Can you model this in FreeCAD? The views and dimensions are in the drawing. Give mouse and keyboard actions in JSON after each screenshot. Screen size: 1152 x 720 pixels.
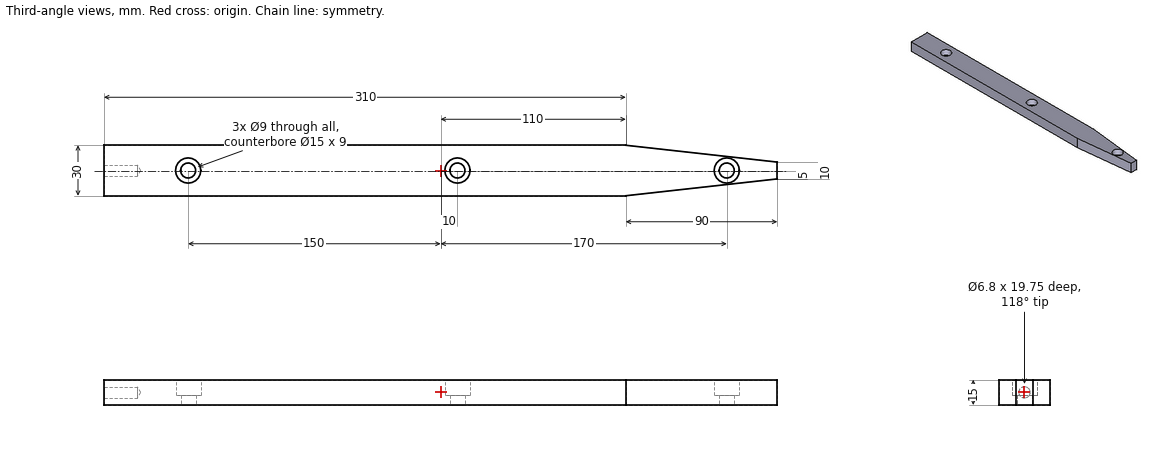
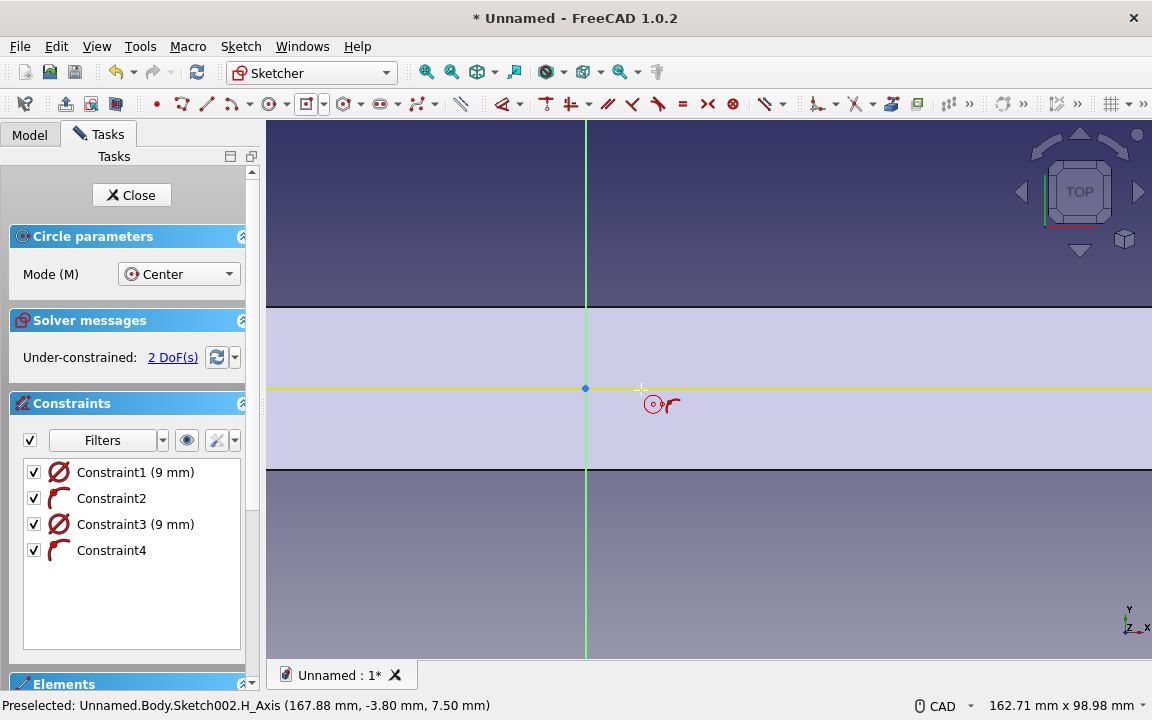
{"action": "scroll", "coordinate": [641, 390], "scroll_direction": "down", "scroll_amount": 6}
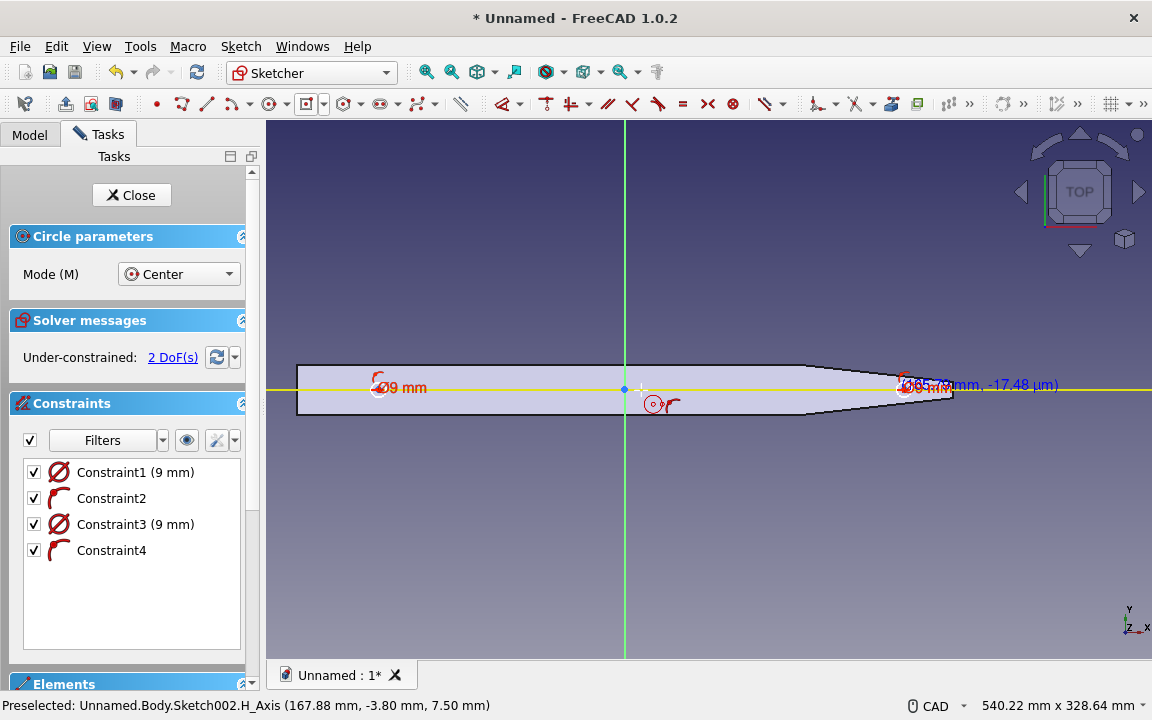
{"action": "left_click", "coordinate": [641, 390]}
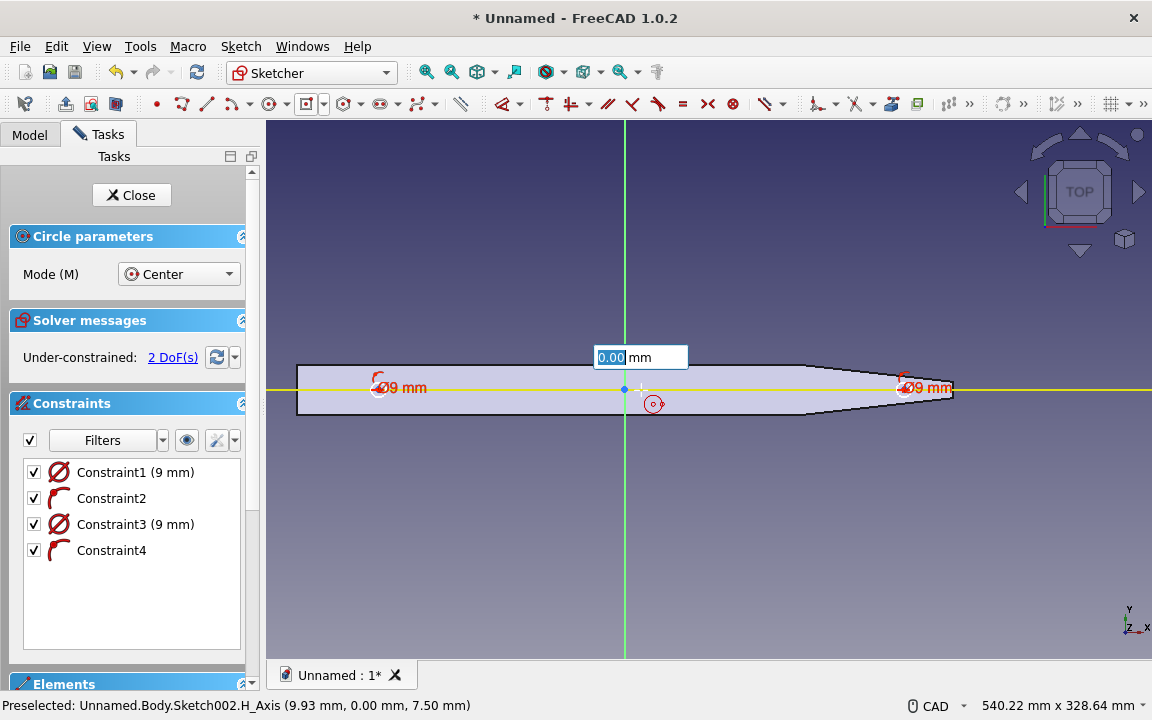
{"action": "scroll", "coordinate": [639, 397], "scroll_direction": "up", "scroll_amount": 5}
{"action": "mouse_move", "coordinate": [637, 396]}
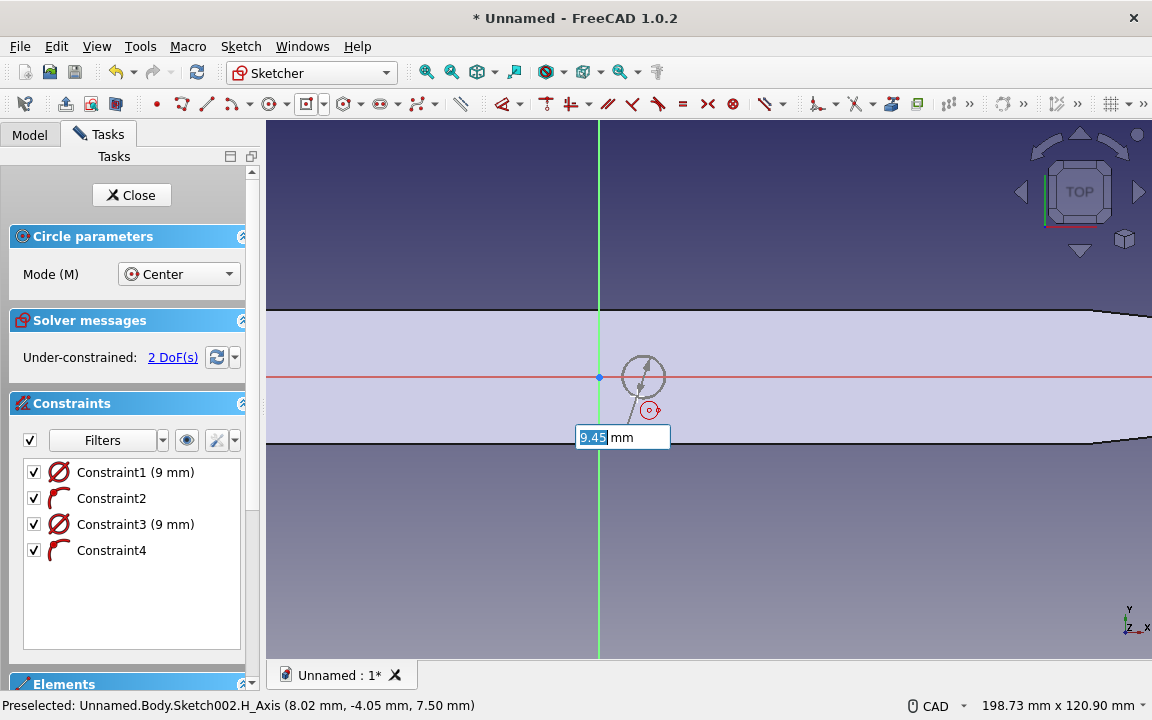
{"action": "type", "text": "9"}
{"action": "key", "text": "Return"}
{"action": "key", "text": "Escape"}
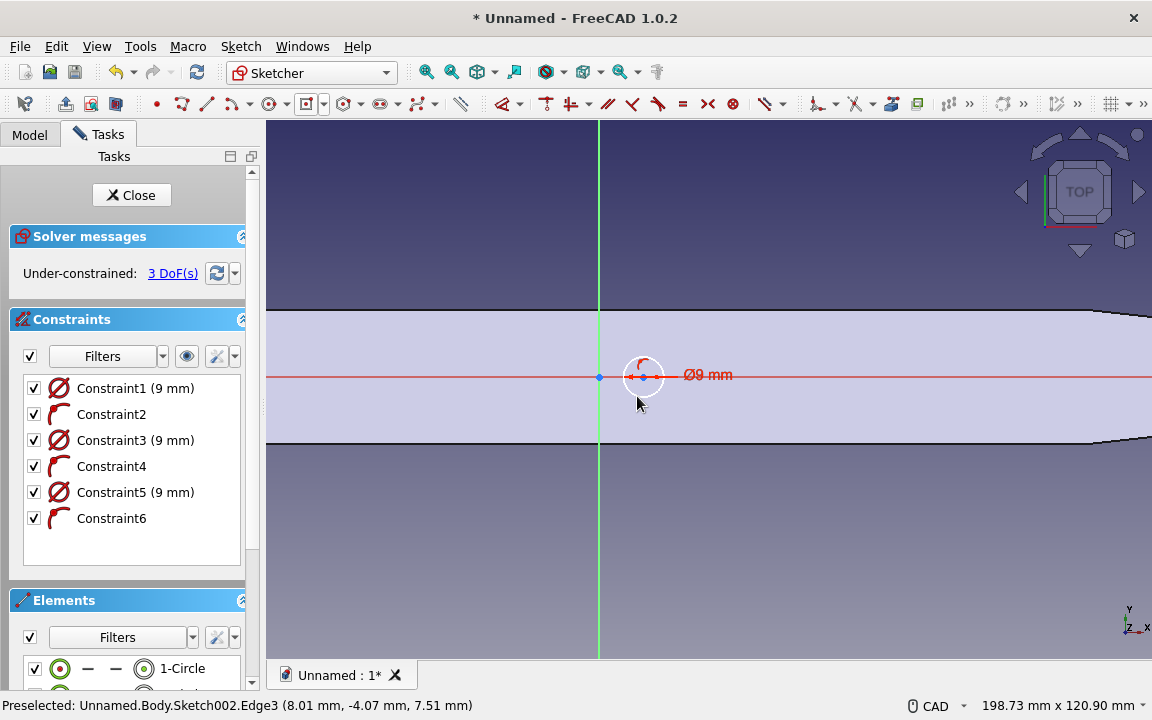
{"action": "key", "text": "d"}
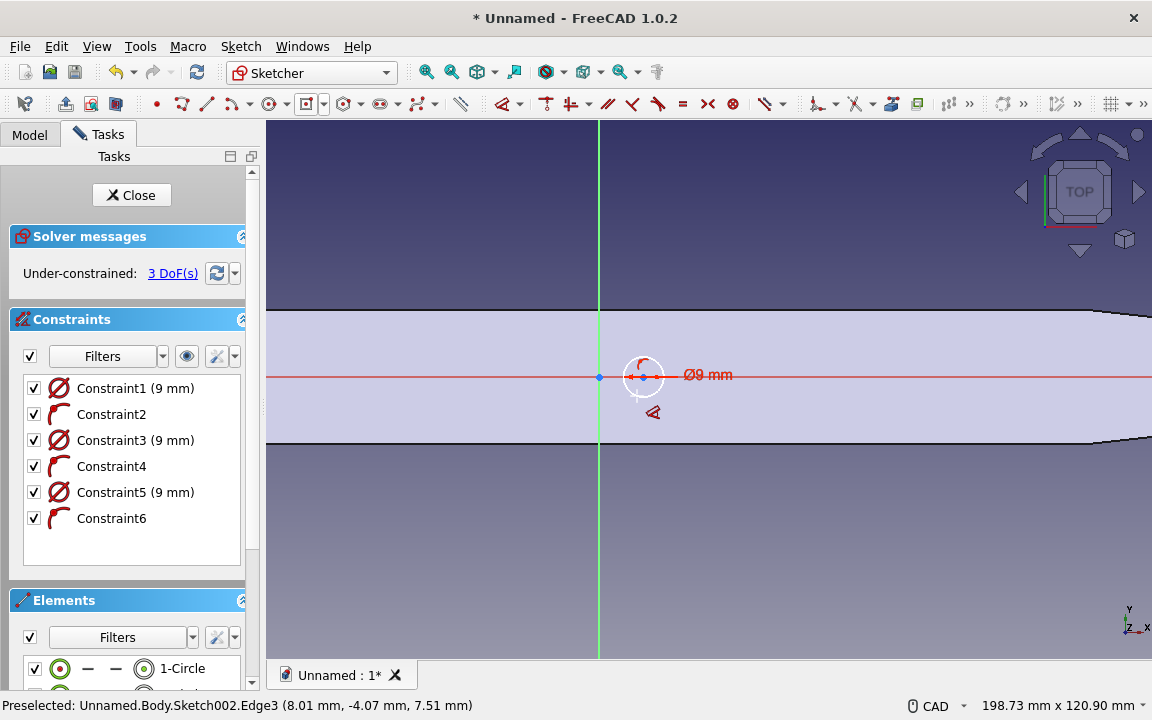
{"action": "left_click", "coordinate": [644, 377]}
{"action": "left_click", "coordinate": [622, 411]}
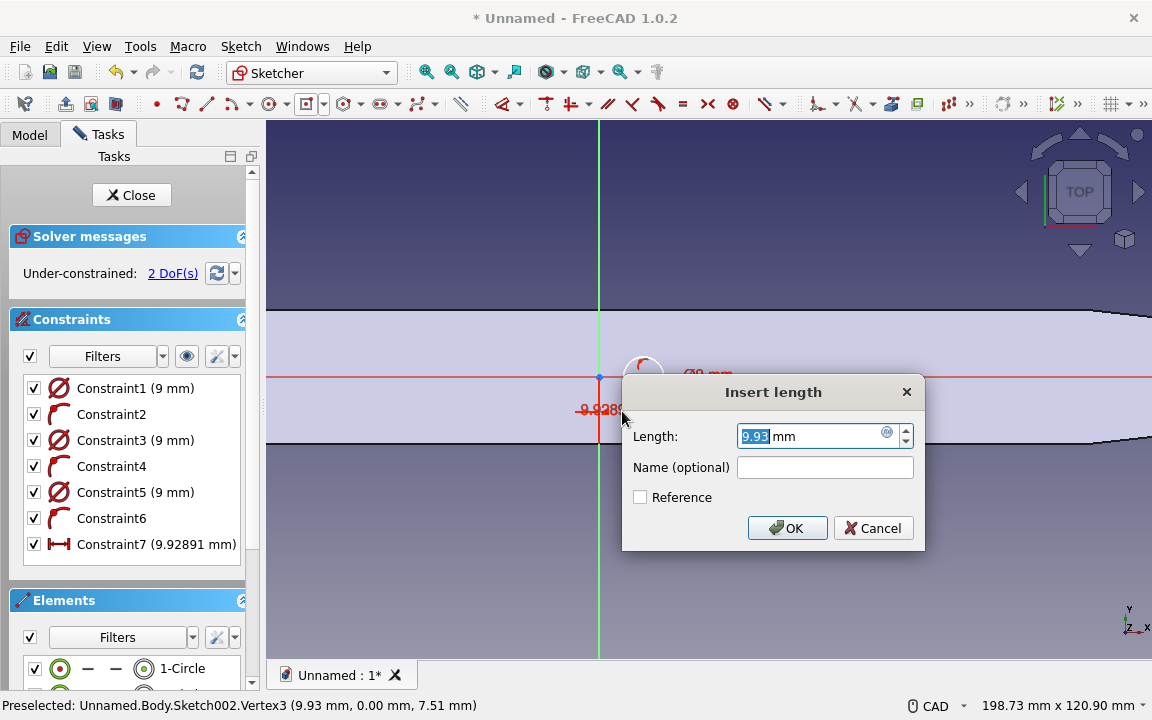
{"action": "type", "text": "10"}
{"action": "key", "text": "Return"}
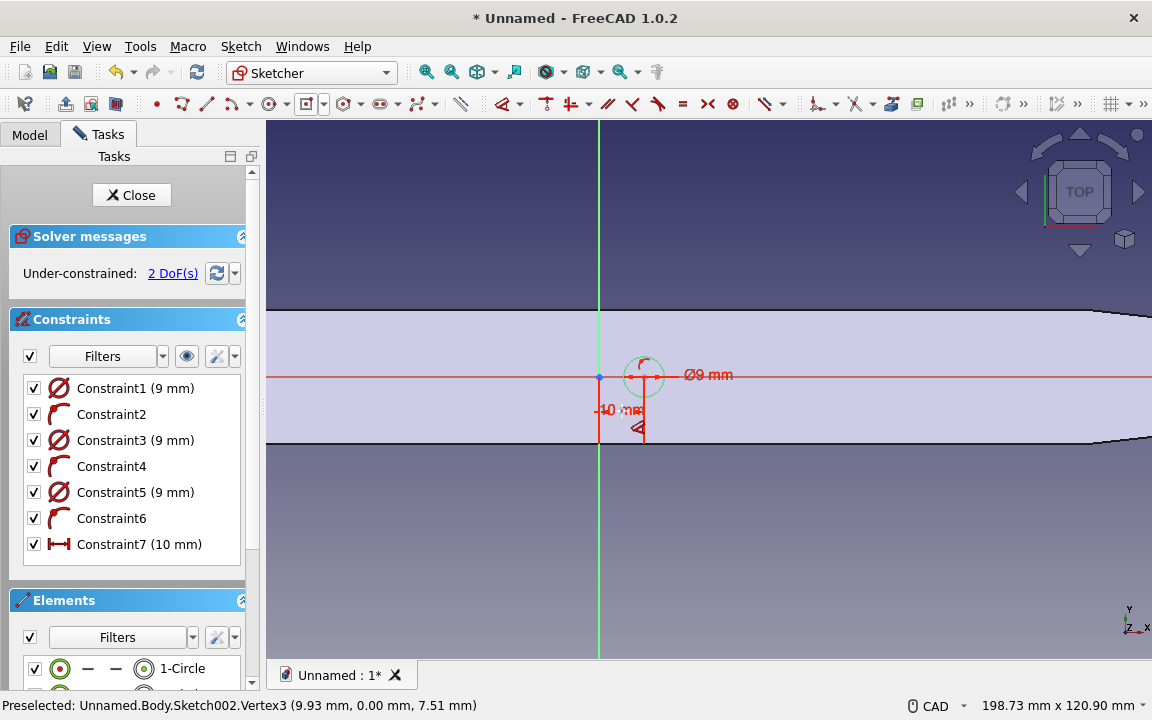
{"action": "scroll", "coordinate": [638, 397], "scroll_direction": "down", "scroll_amount": 5}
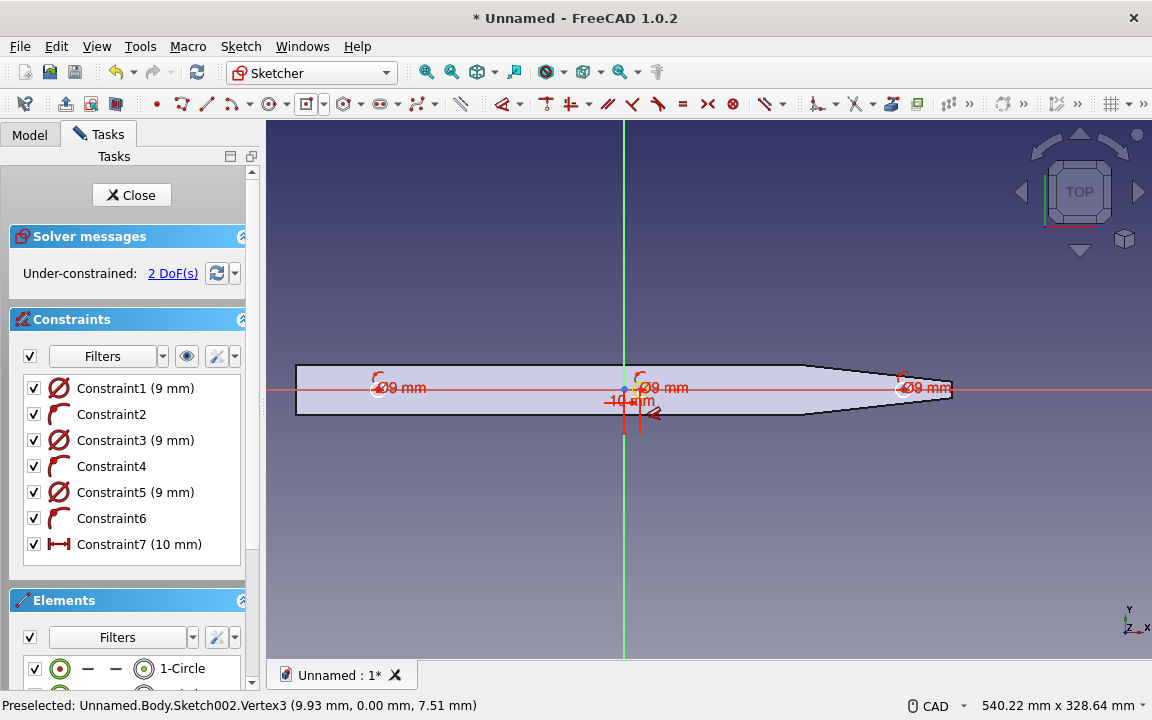
{"action": "left_click", "coordinate": [378, 390]}
{"action": "left_click", "coordinate": [501, 424]}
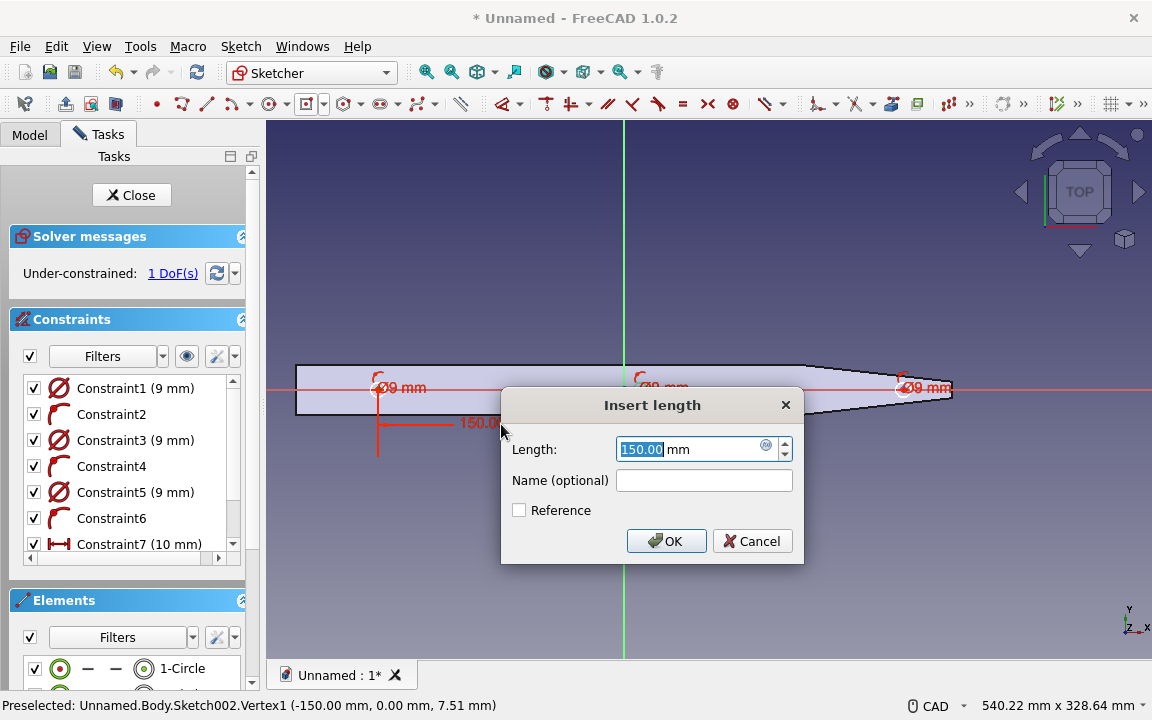
{"action": "type", "text": "150"}
{"action": "key", "text": "Return"}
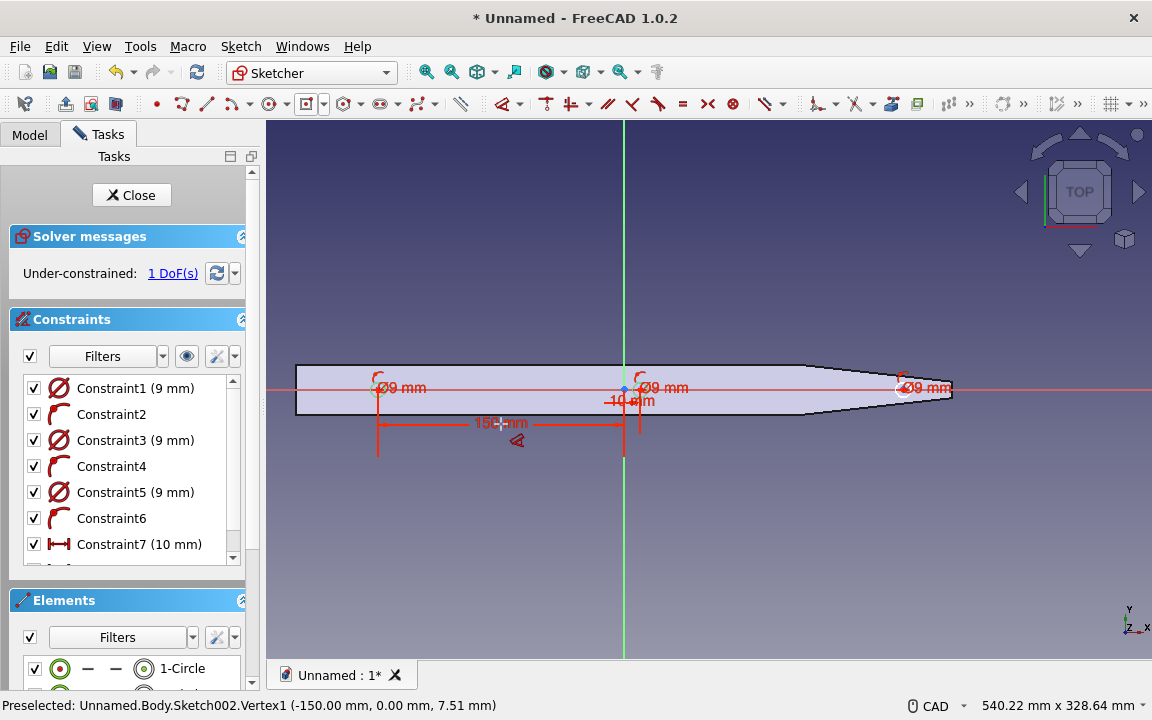
{"action": "left_click", "coordinate": [903, 390]}
{"action": "left_click", "coordinate": [764, 424]}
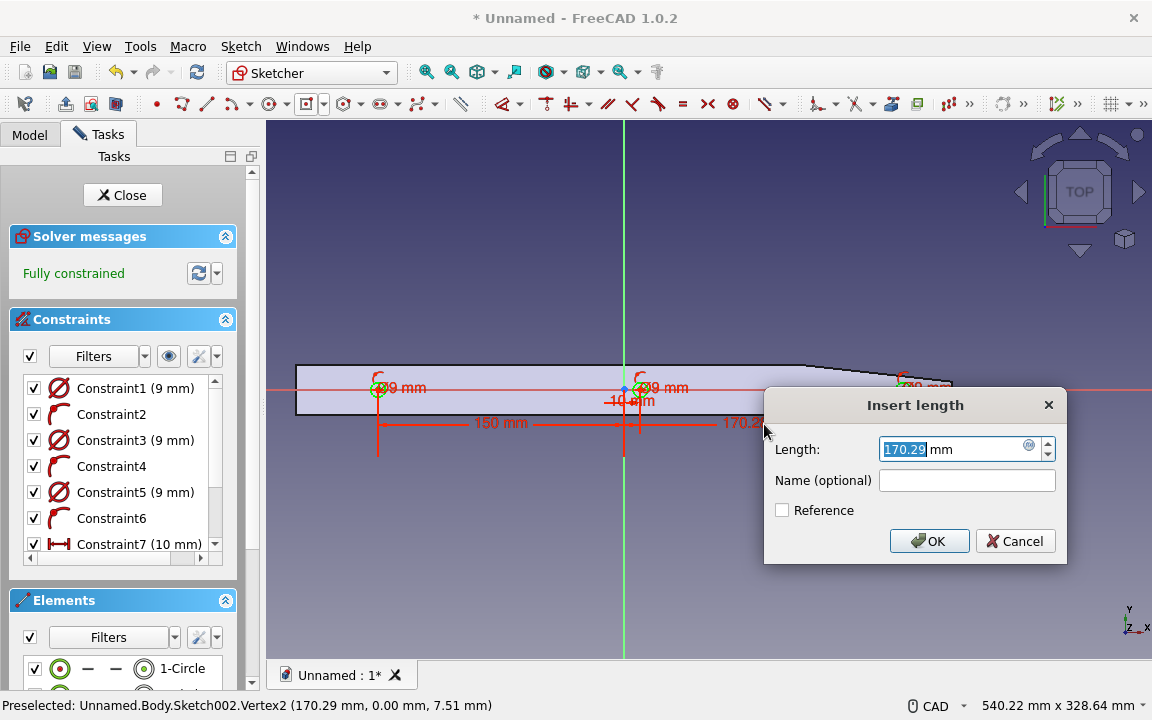
{"action": "type", "text": "170"}
{"action": "key", "text": "Return"}
{"action": "key", "text": "Escape"}